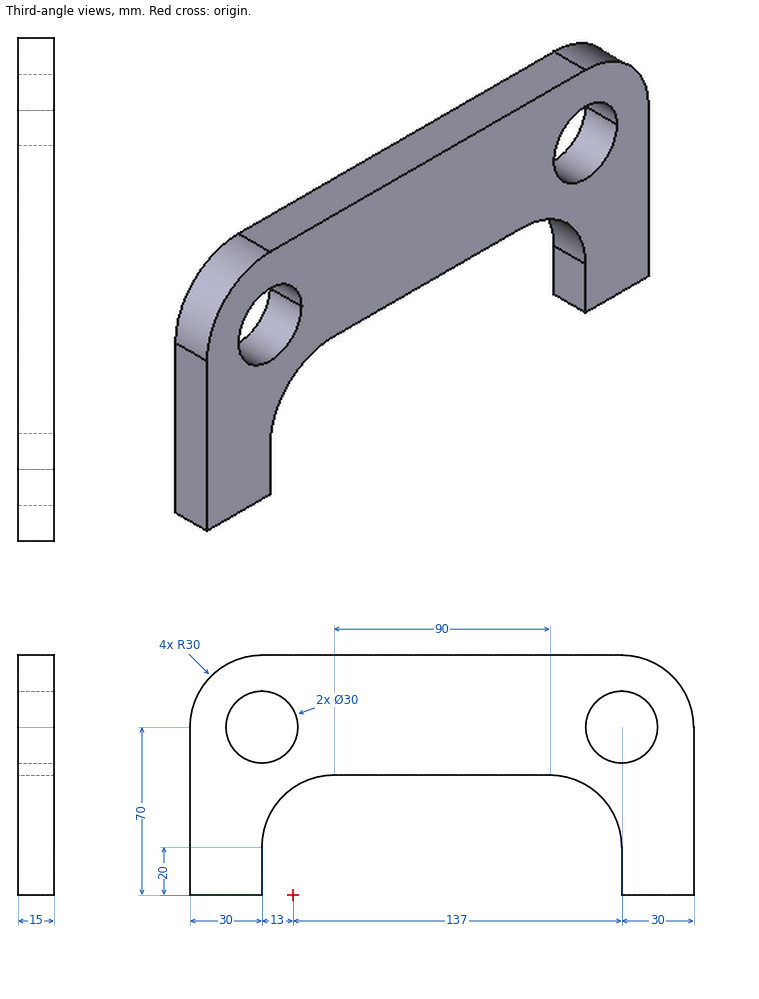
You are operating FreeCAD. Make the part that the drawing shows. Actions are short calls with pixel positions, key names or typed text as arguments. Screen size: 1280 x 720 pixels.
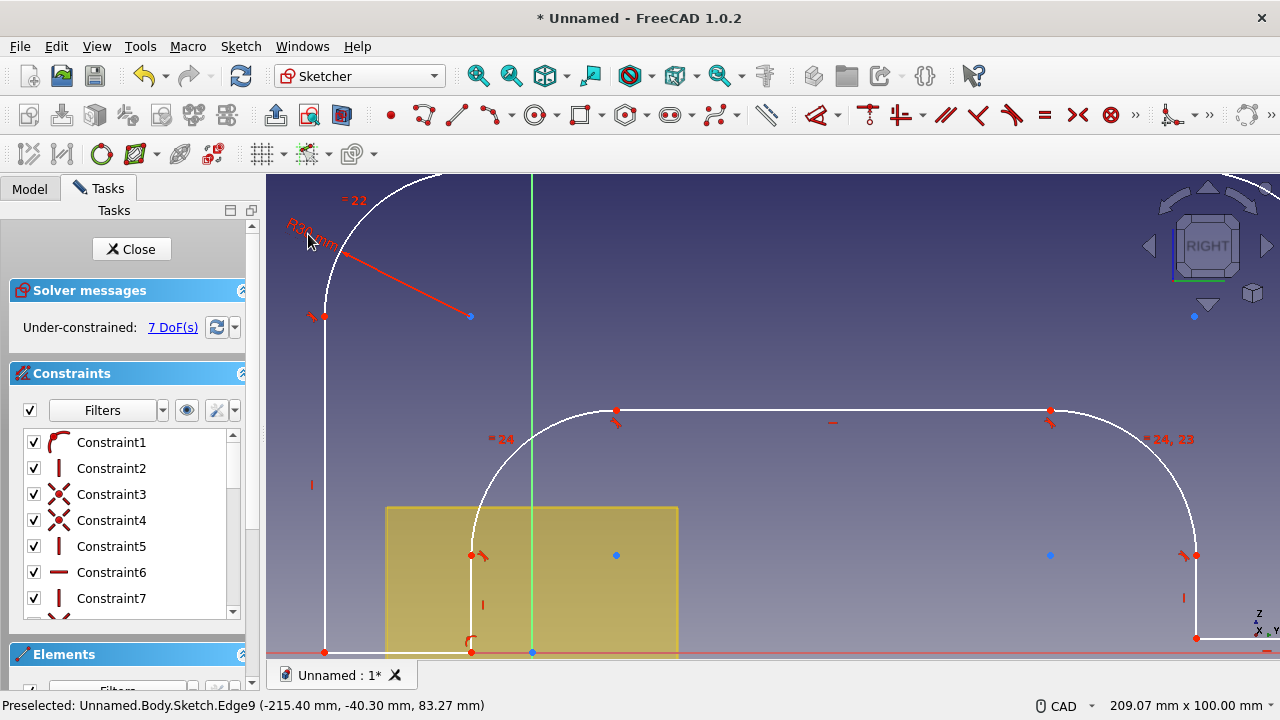
scroll(548, 424, down, 3)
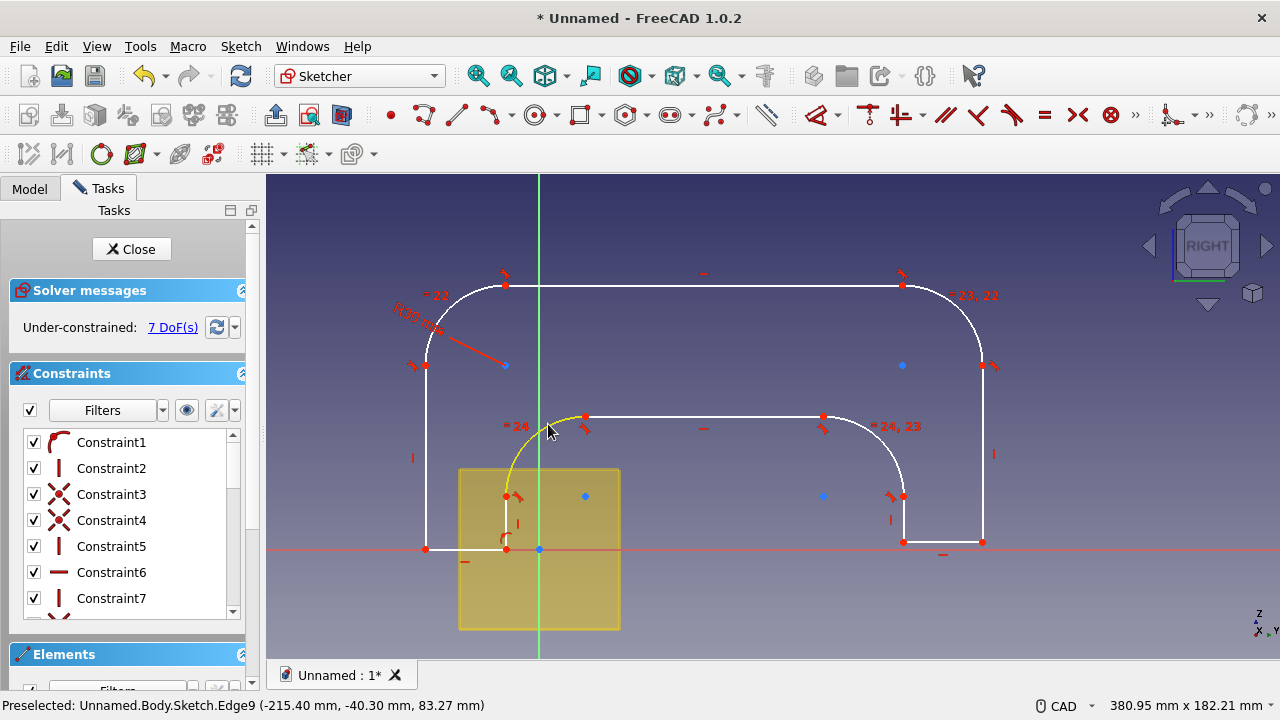
click(983, 542)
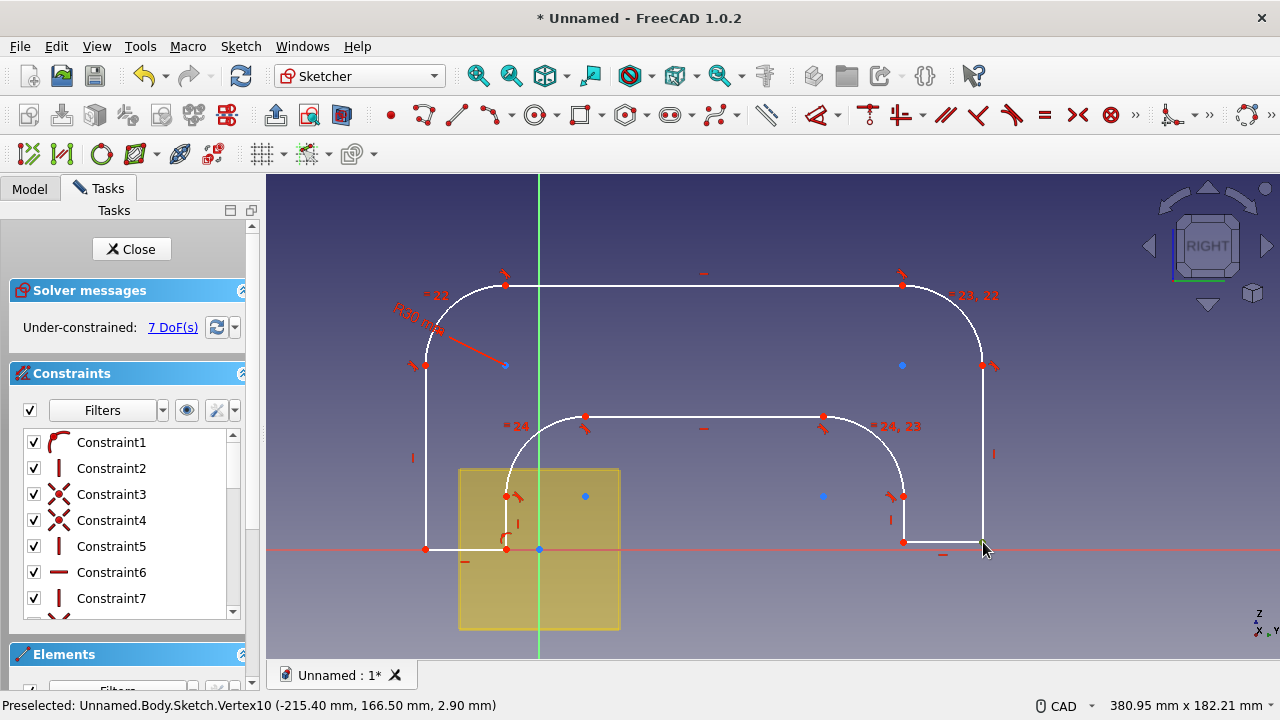
click(353, 550)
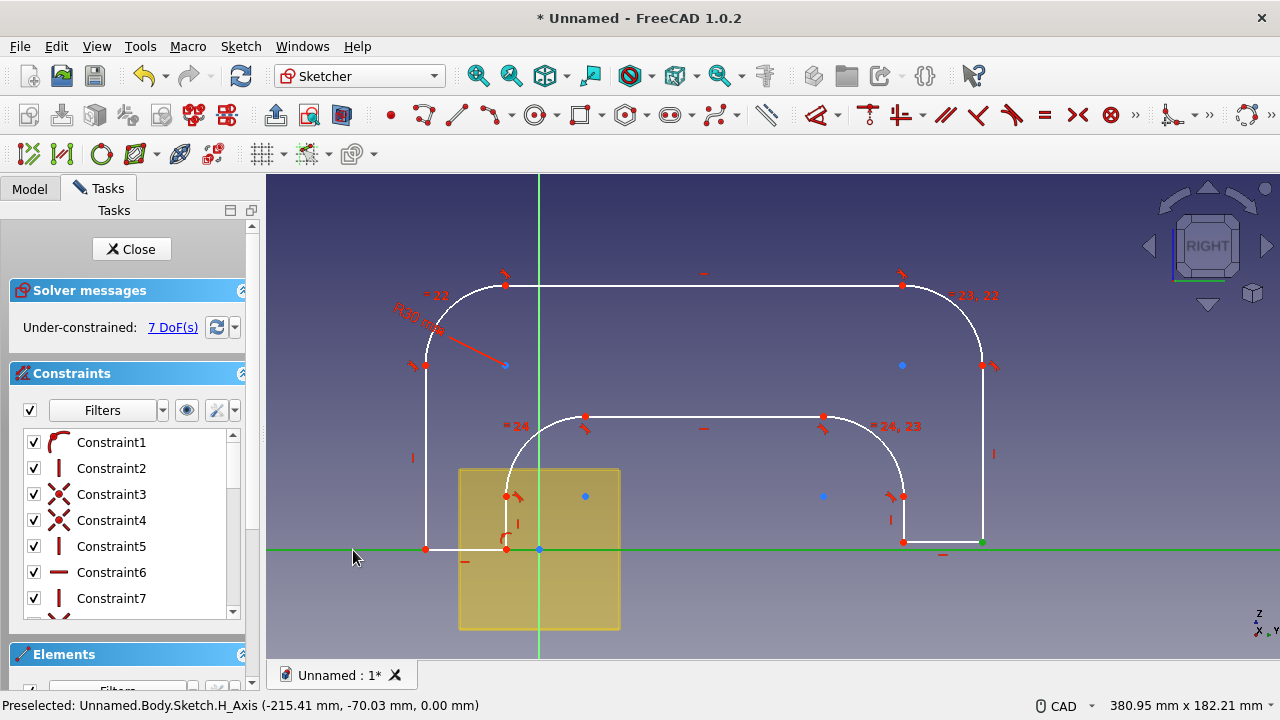
key(c)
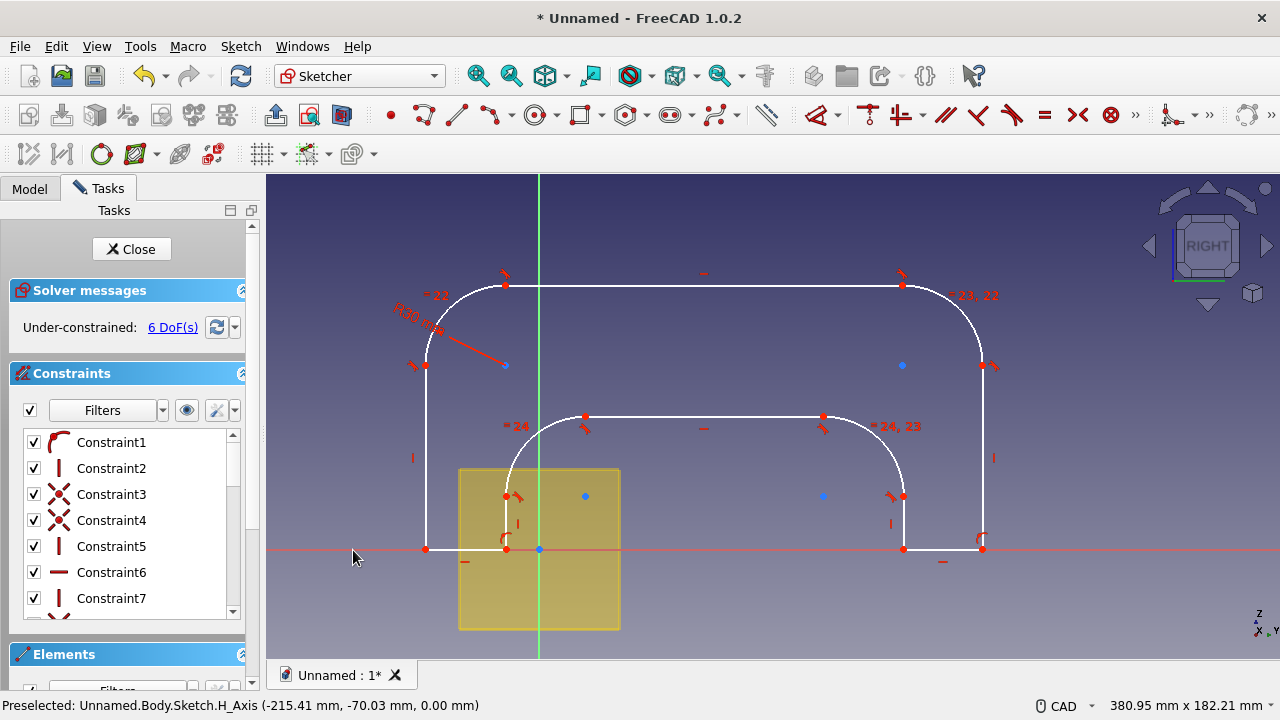
key(d)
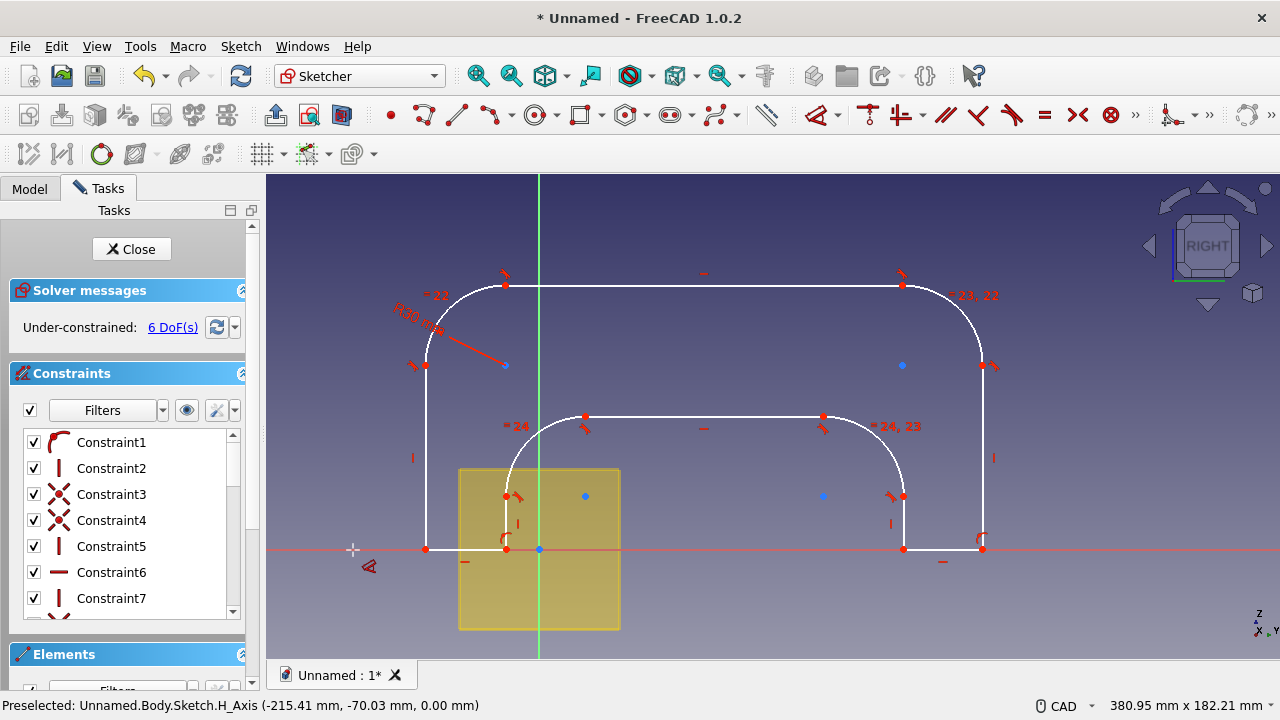
click(506, 513)
click(472, 523)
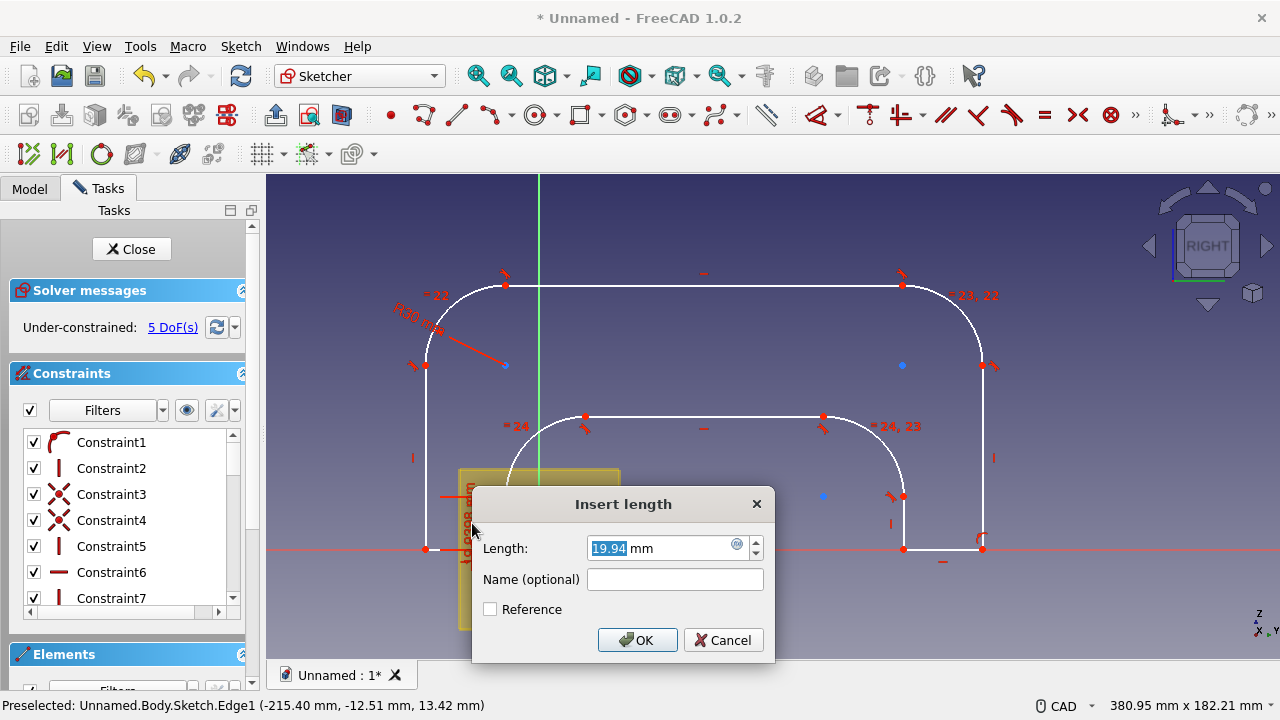
text(20)
key(Return)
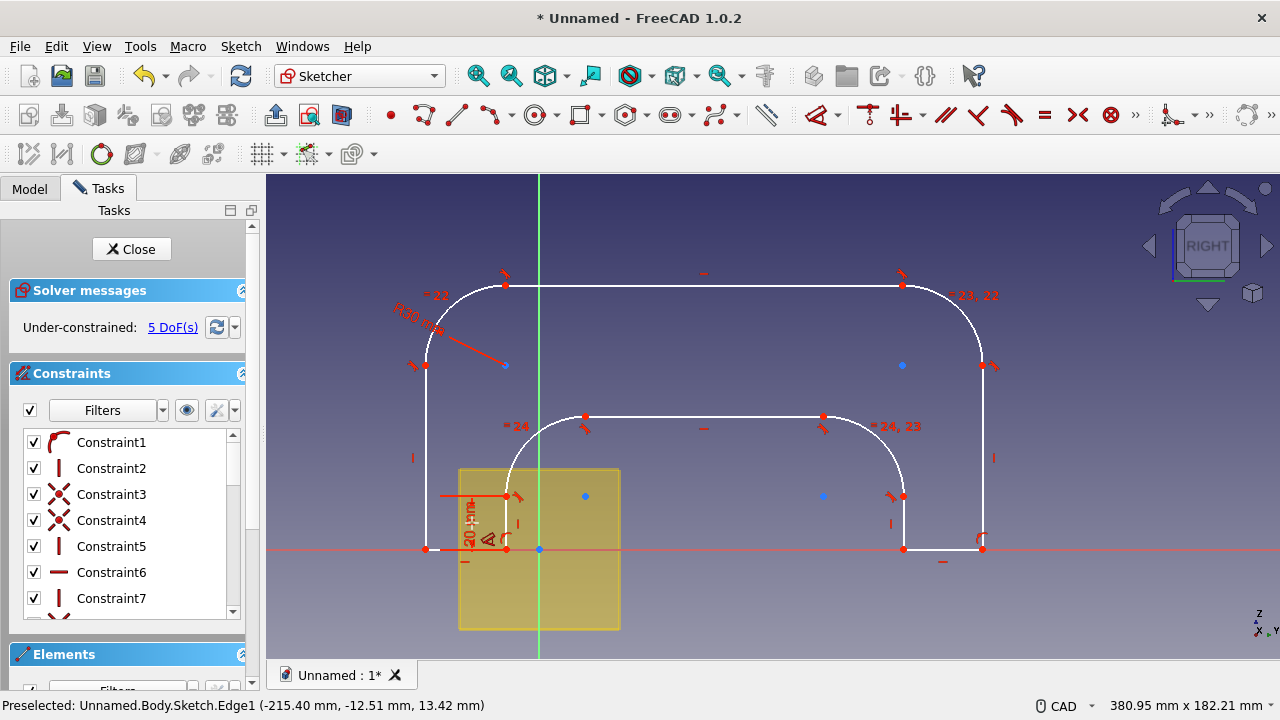
click(482, 550)
click(466, 584)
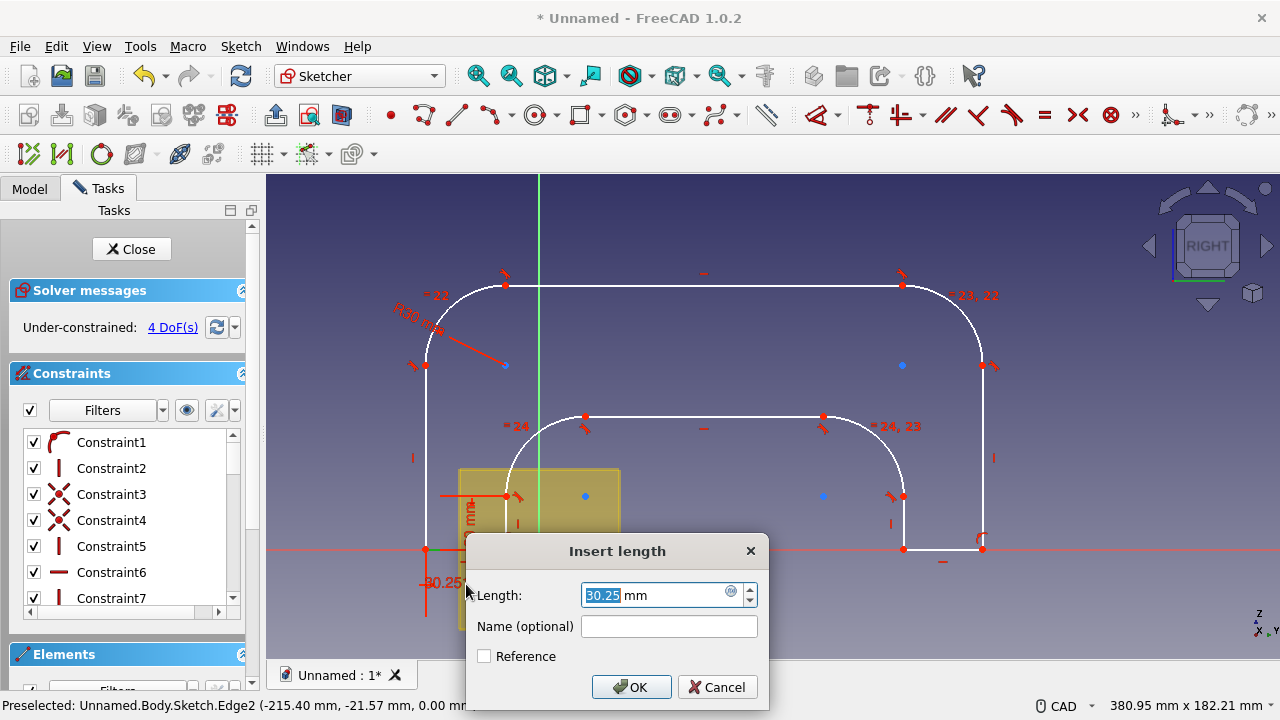
text(30)
key(Return)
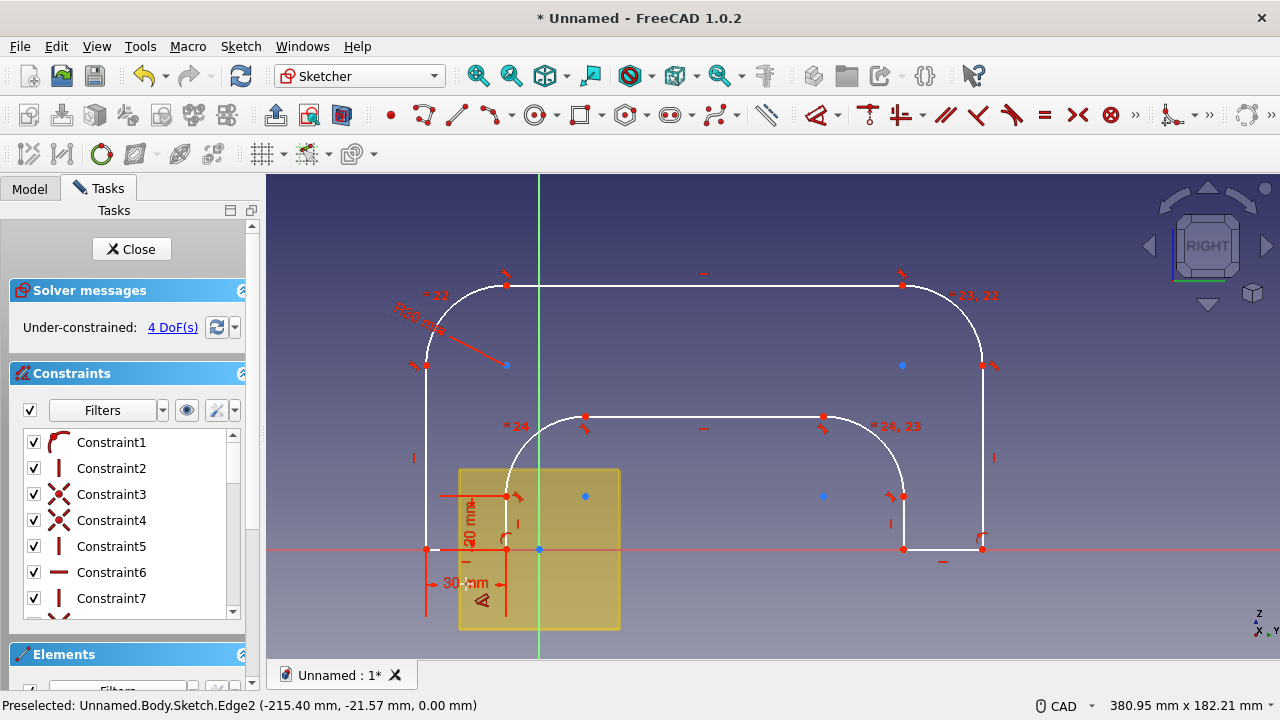
click(426, 494)
click(392, 458)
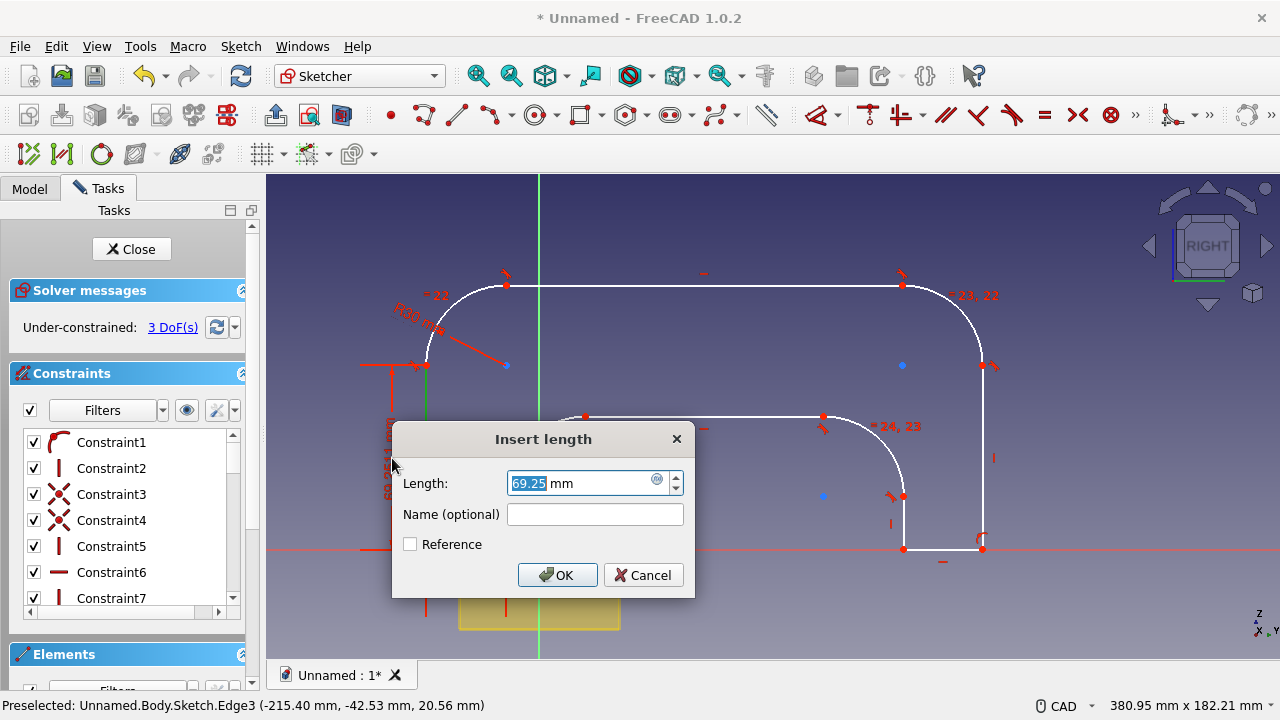
text(70)
key(Return)